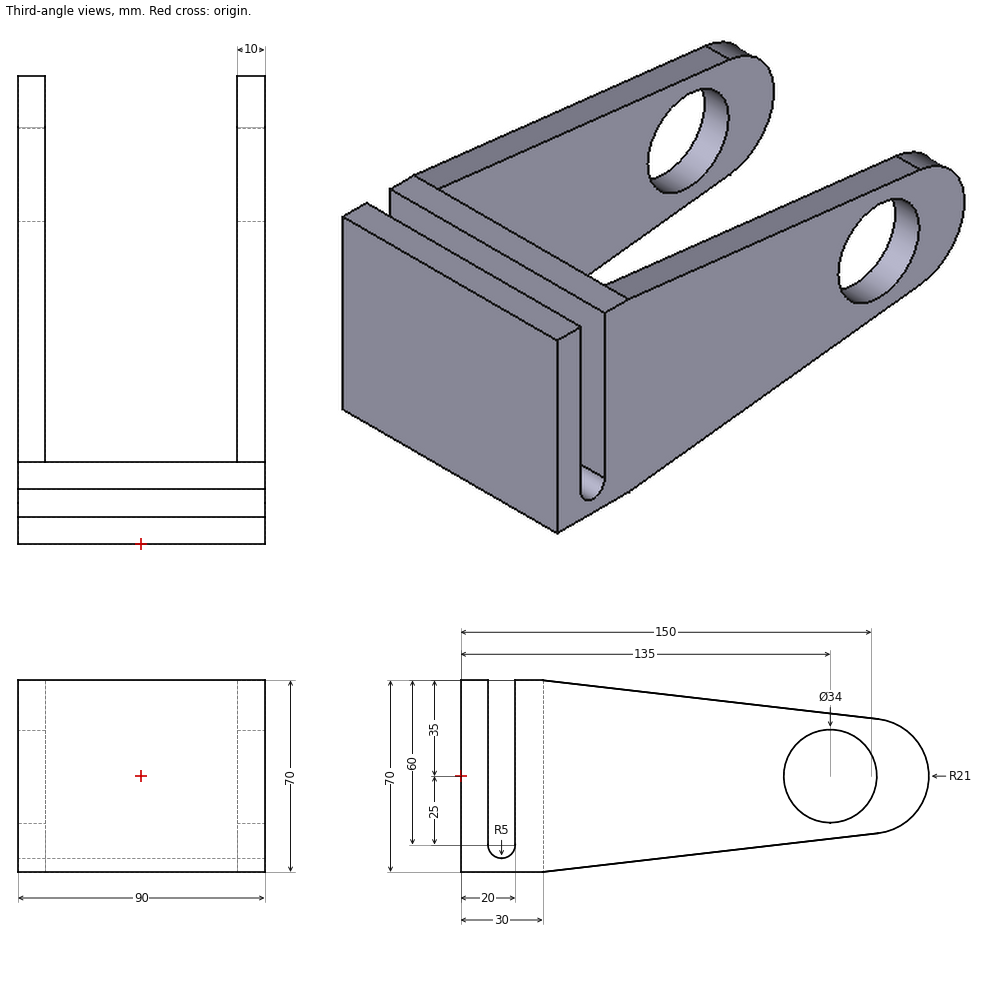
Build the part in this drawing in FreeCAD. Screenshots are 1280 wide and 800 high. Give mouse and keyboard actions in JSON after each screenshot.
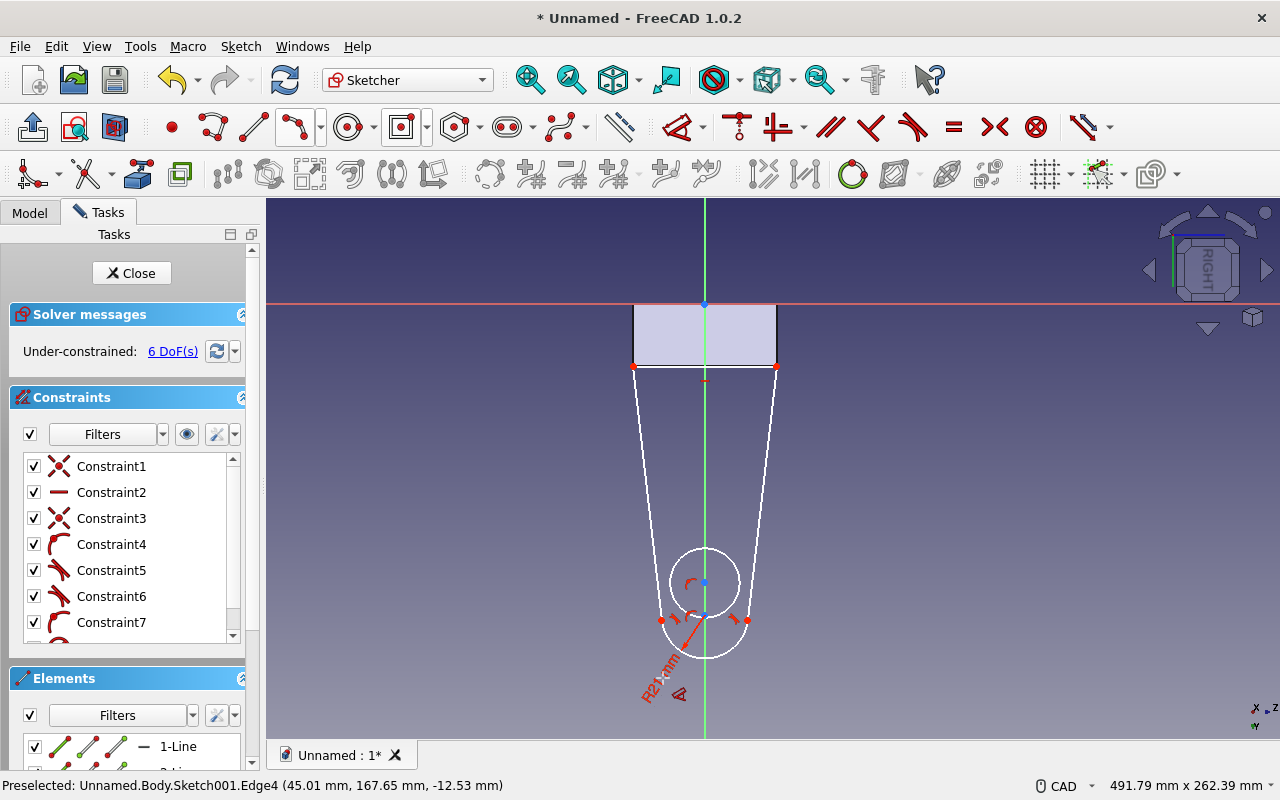
{"action": "left_click", "coordinate": [729, 558]}
{"action": "left_click", "coordinate": [769, 563]}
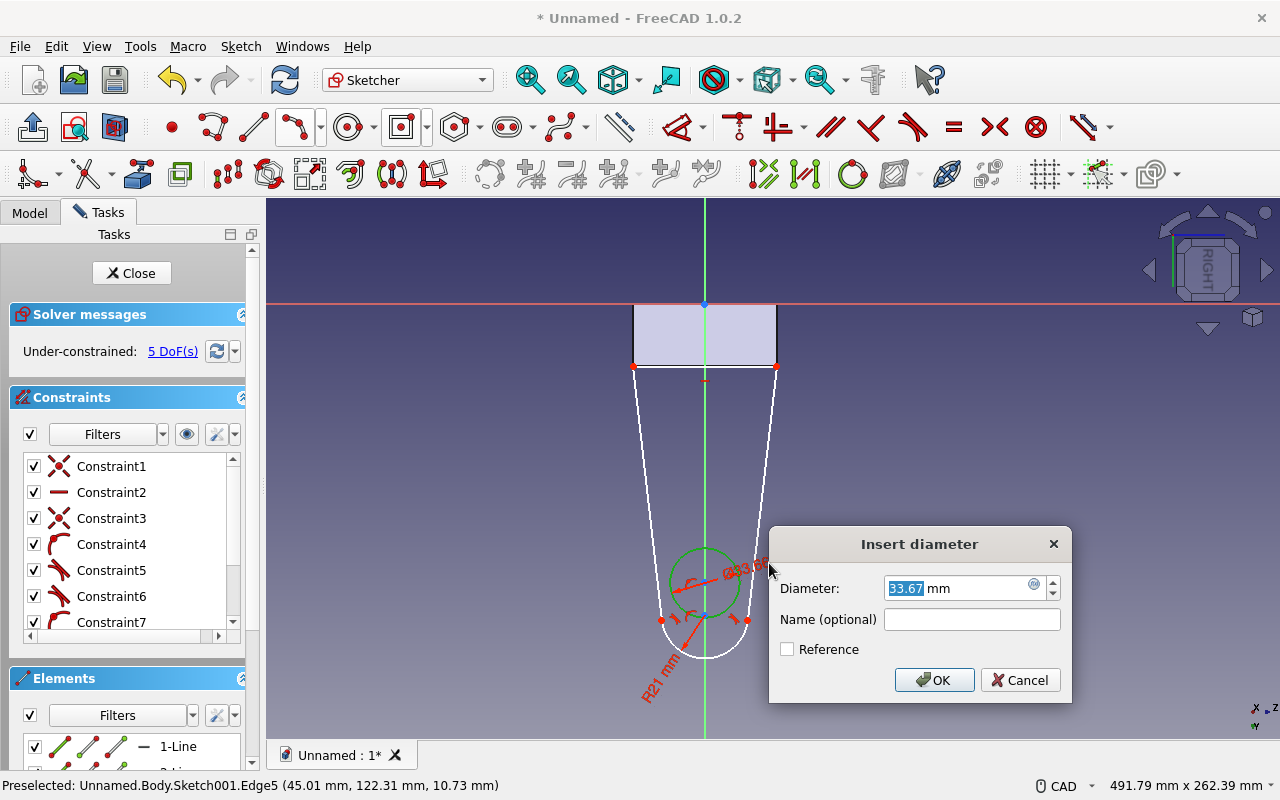
{"action": "type", "text": "34"}
{"action": "key", "text": "Return"}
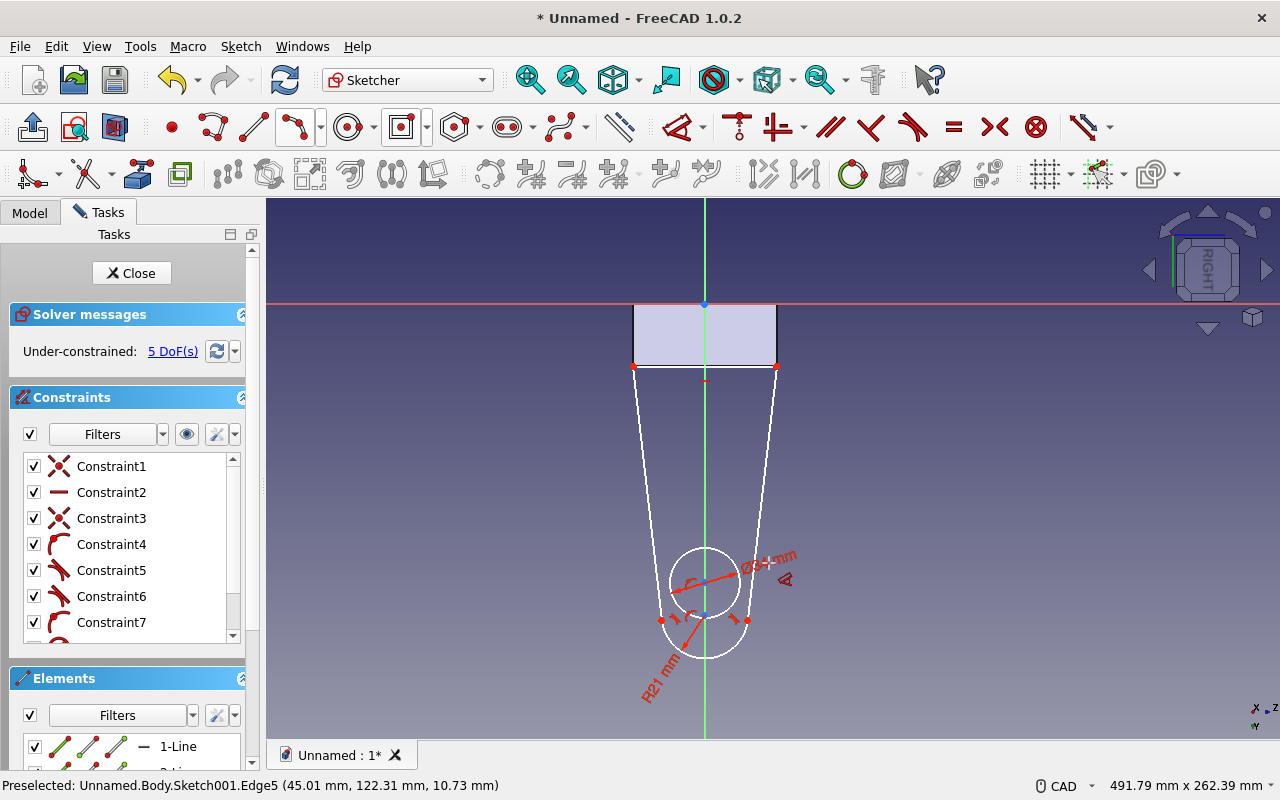
{"action": "left_click", "coordinate": [734, 367]}
{"action": "left_click", "coordinate": [672, 333]}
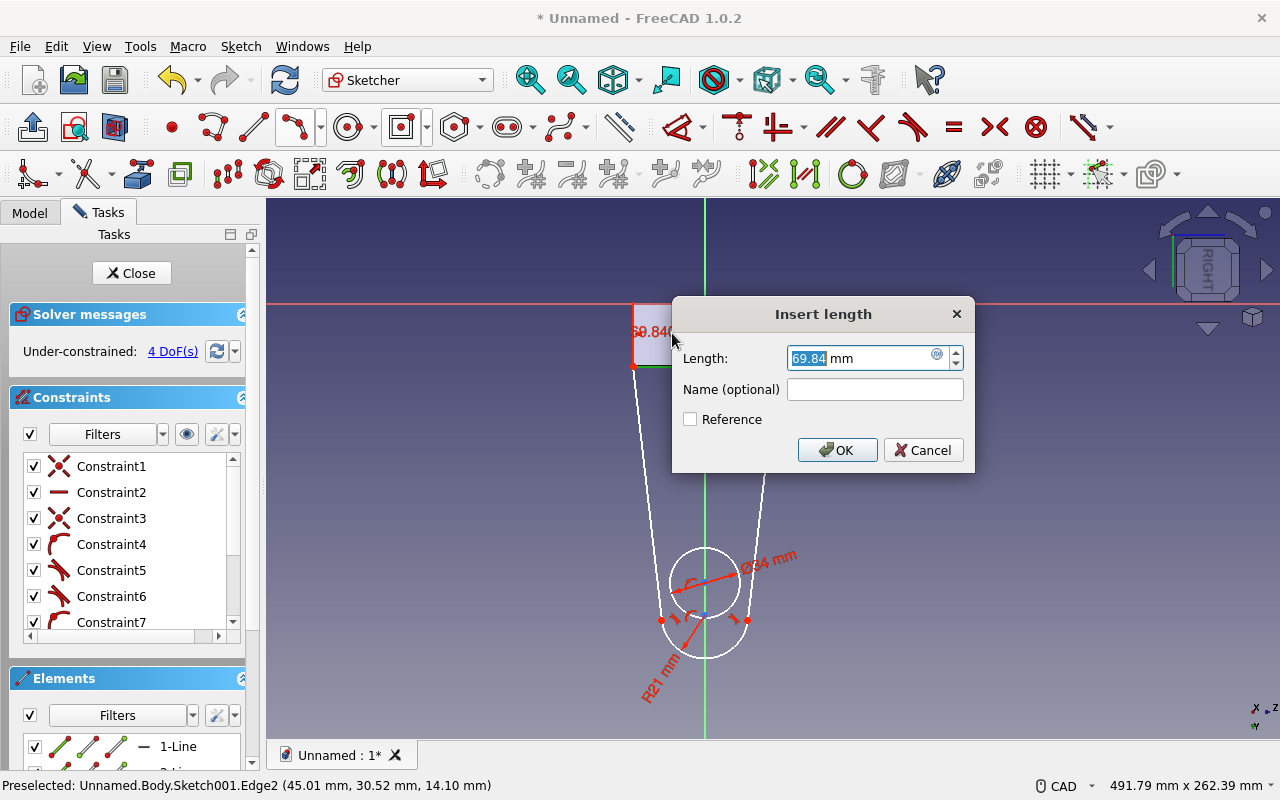
{"action": "type", "text": "70"}
{"action": "key", "text": "Return"}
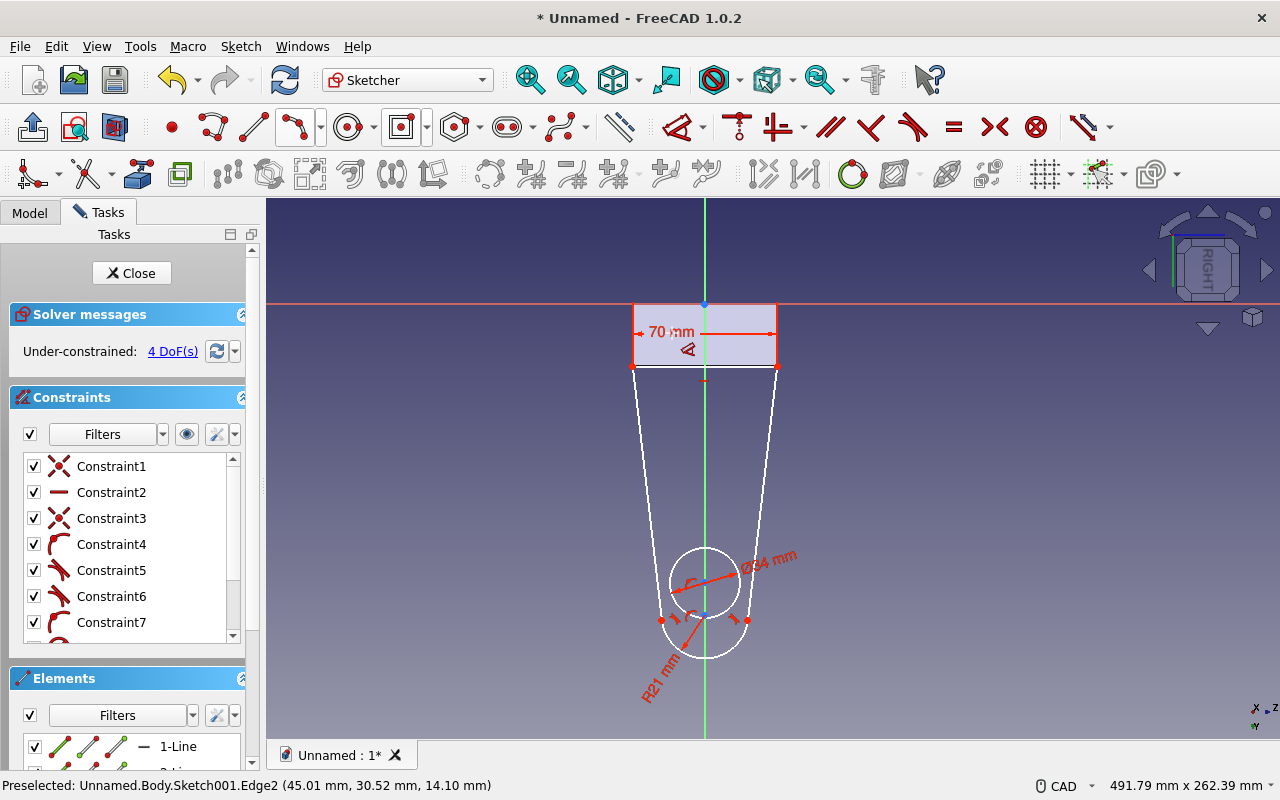
{"action": "left_click", "coordinate": [777, 367]}
{"action": "left_click", "coordinate": [741, 270]}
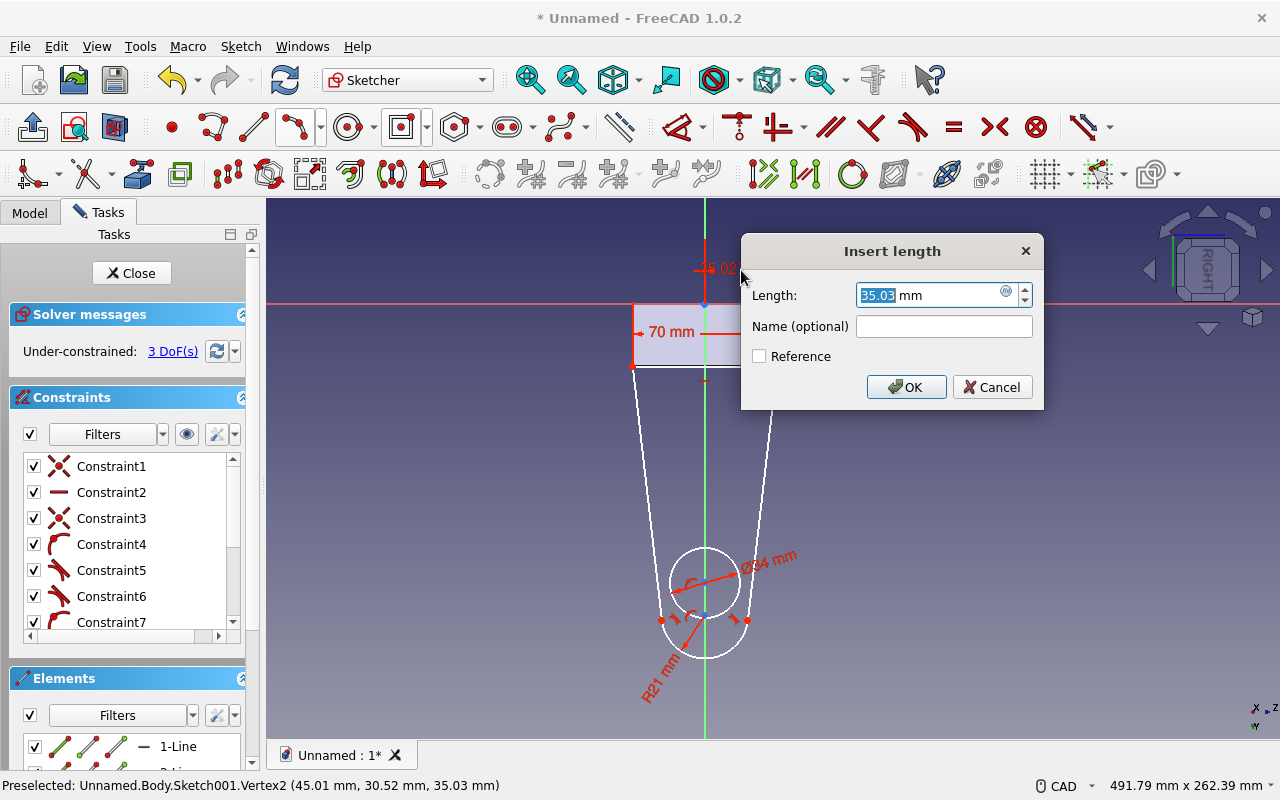
{"action": "type", "text": "35"}
{"action": "key", "text": "Return"}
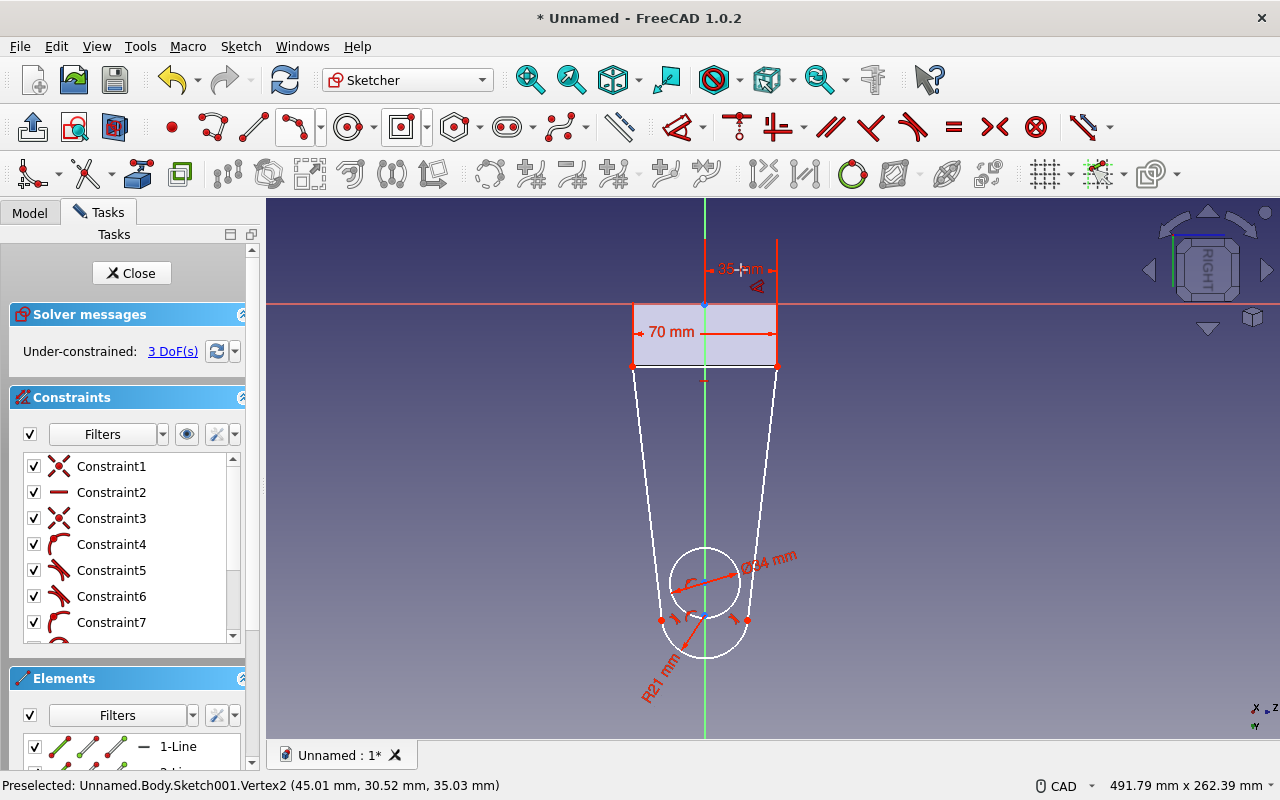
{"action": "left_click", "coordinate": [777, 367]}
{"action": "left_click", "coordinate": [811, 336]}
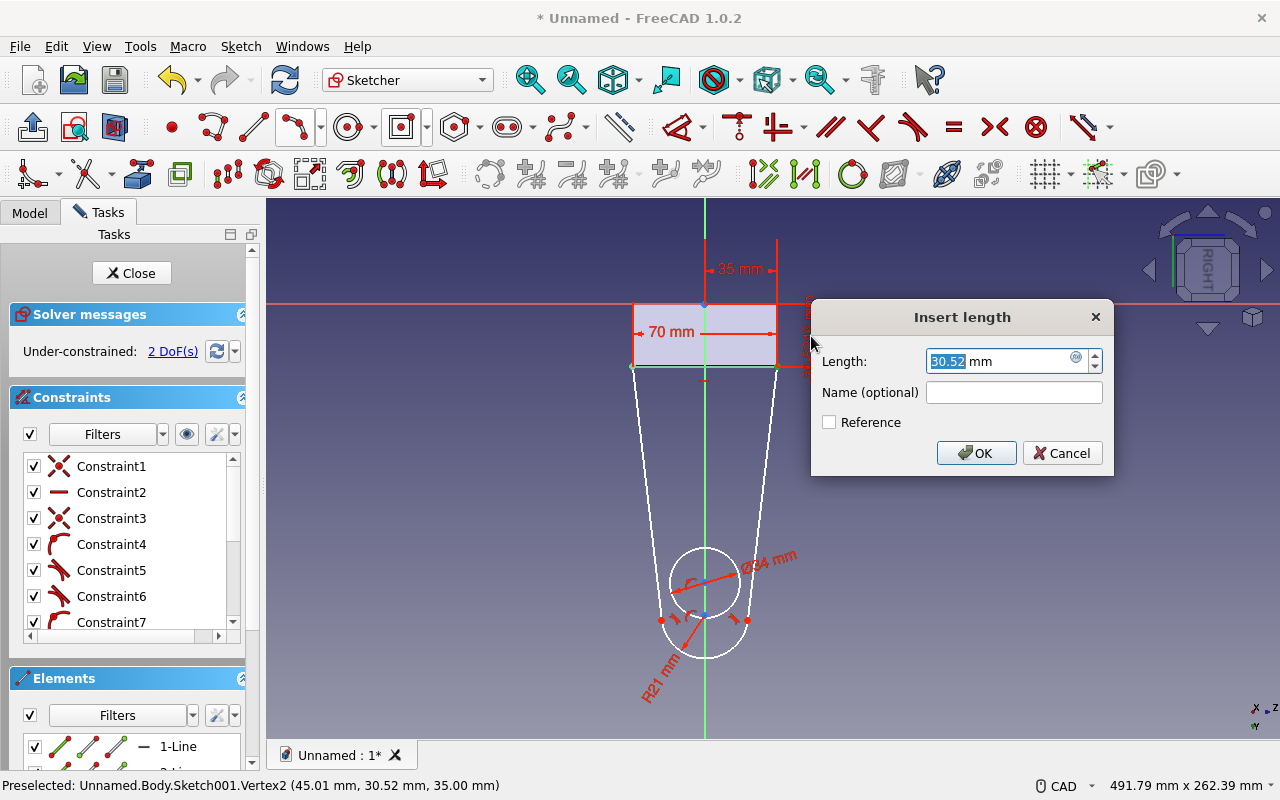
{"action": "type", "text": "30"}
{"action": "key", "text": "Return"}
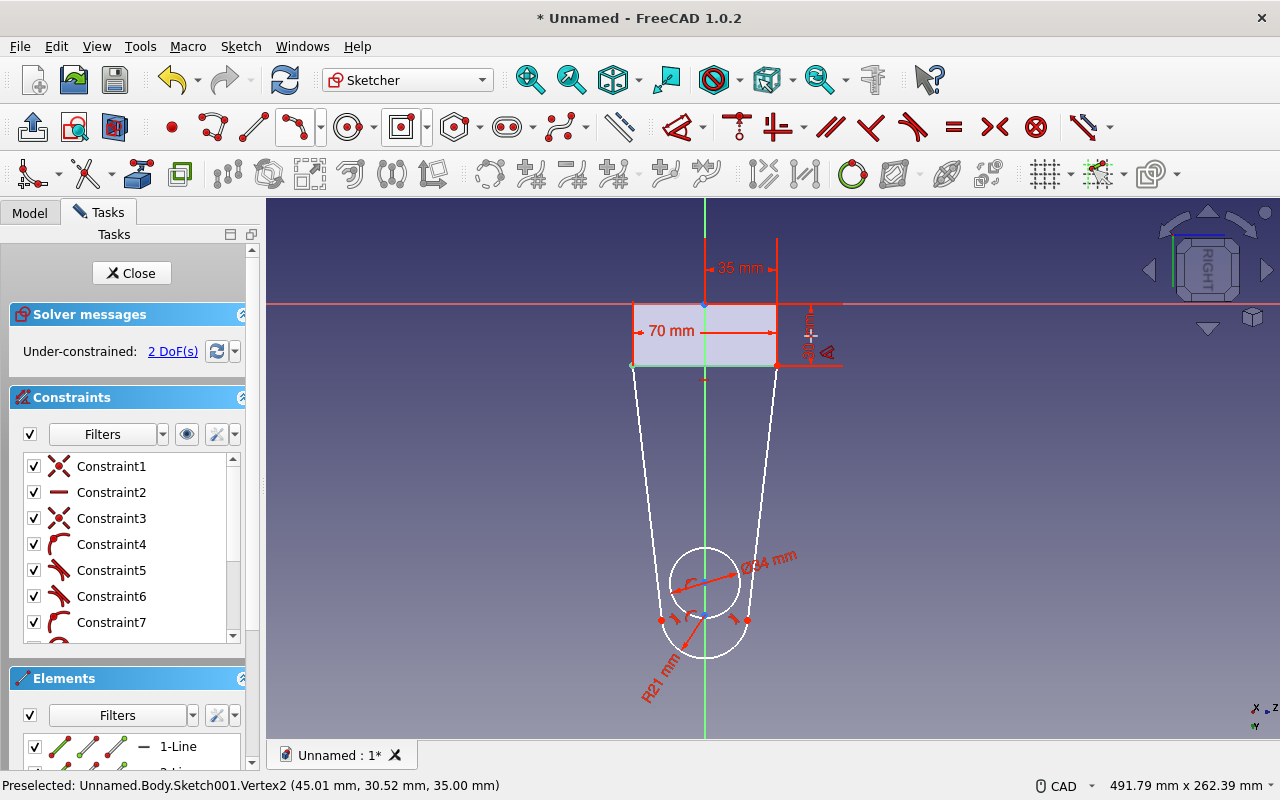
{"action": "left_click", "coordinate": [705, 583]}
{"action": "left_click", "coordinate": [739, 444]}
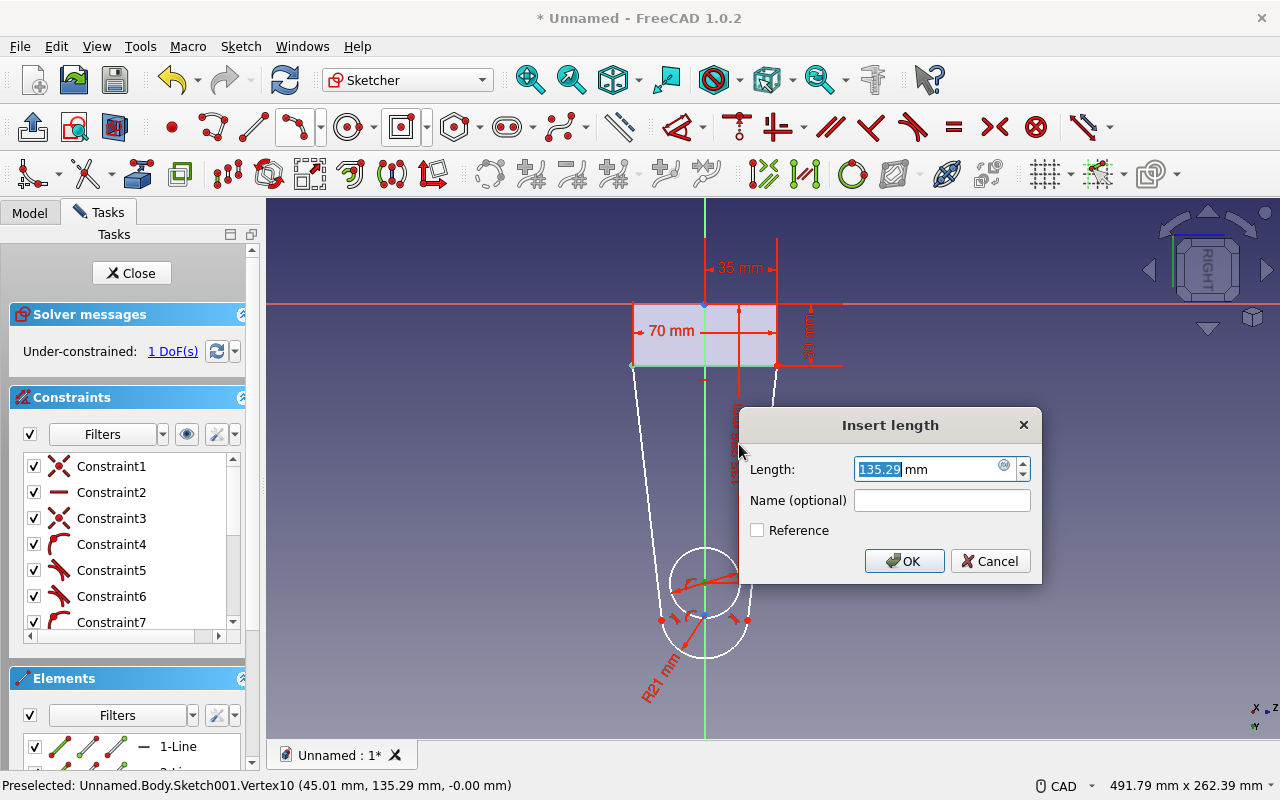
{"action": "type", "text": "135"}
{"action": "key", "text": "Return"}